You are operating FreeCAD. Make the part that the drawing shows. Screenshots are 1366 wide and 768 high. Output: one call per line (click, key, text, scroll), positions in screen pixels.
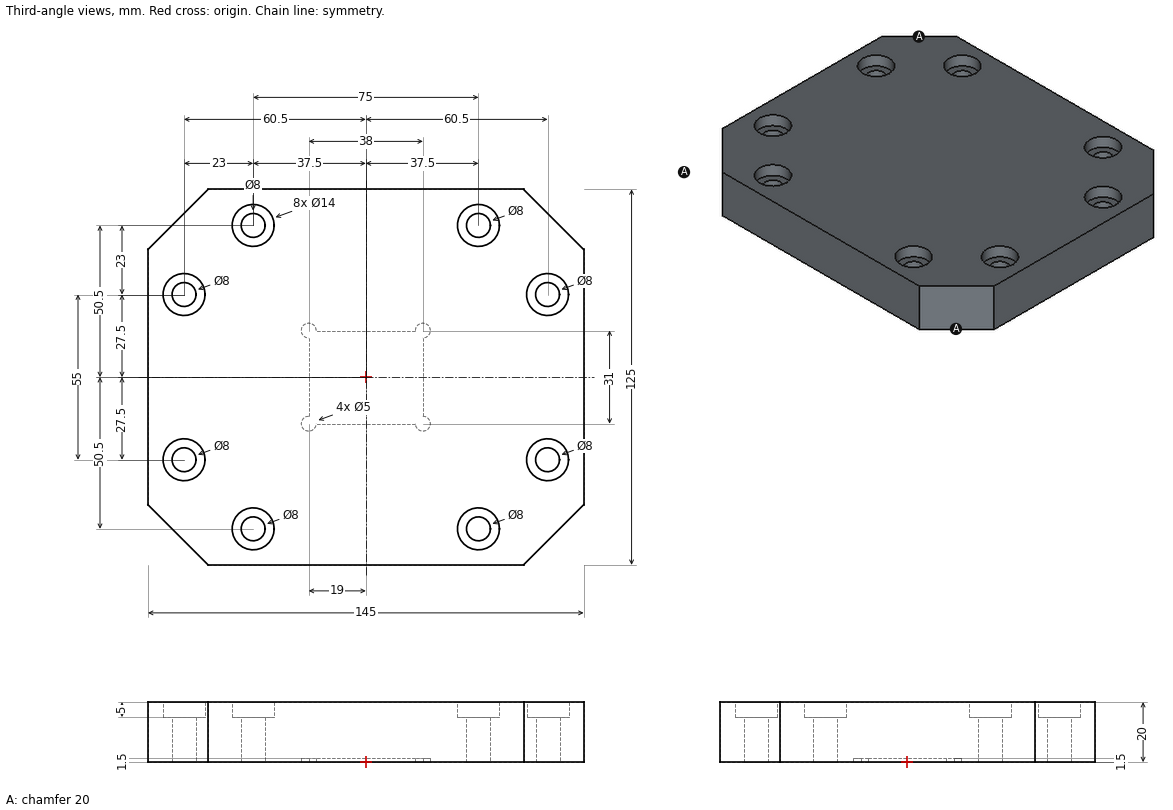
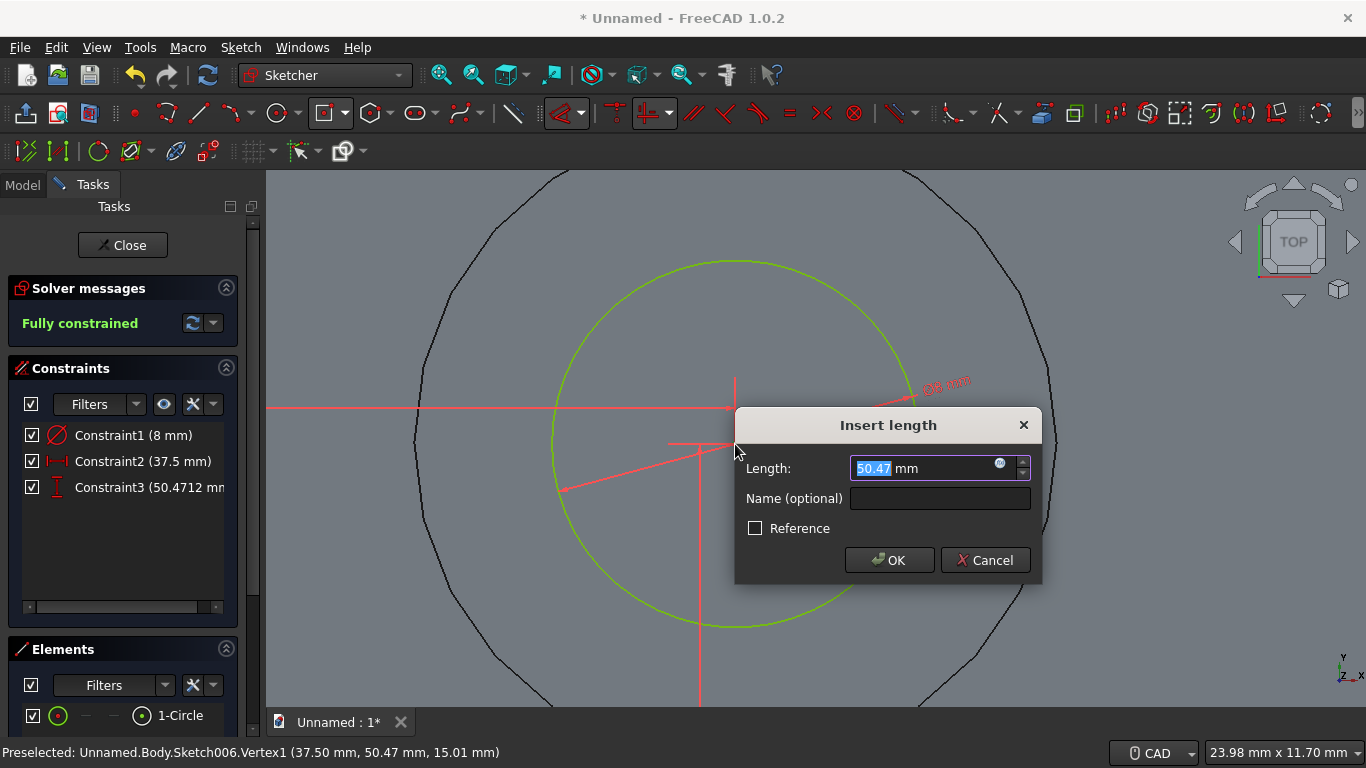
text(50.5)
key(Return)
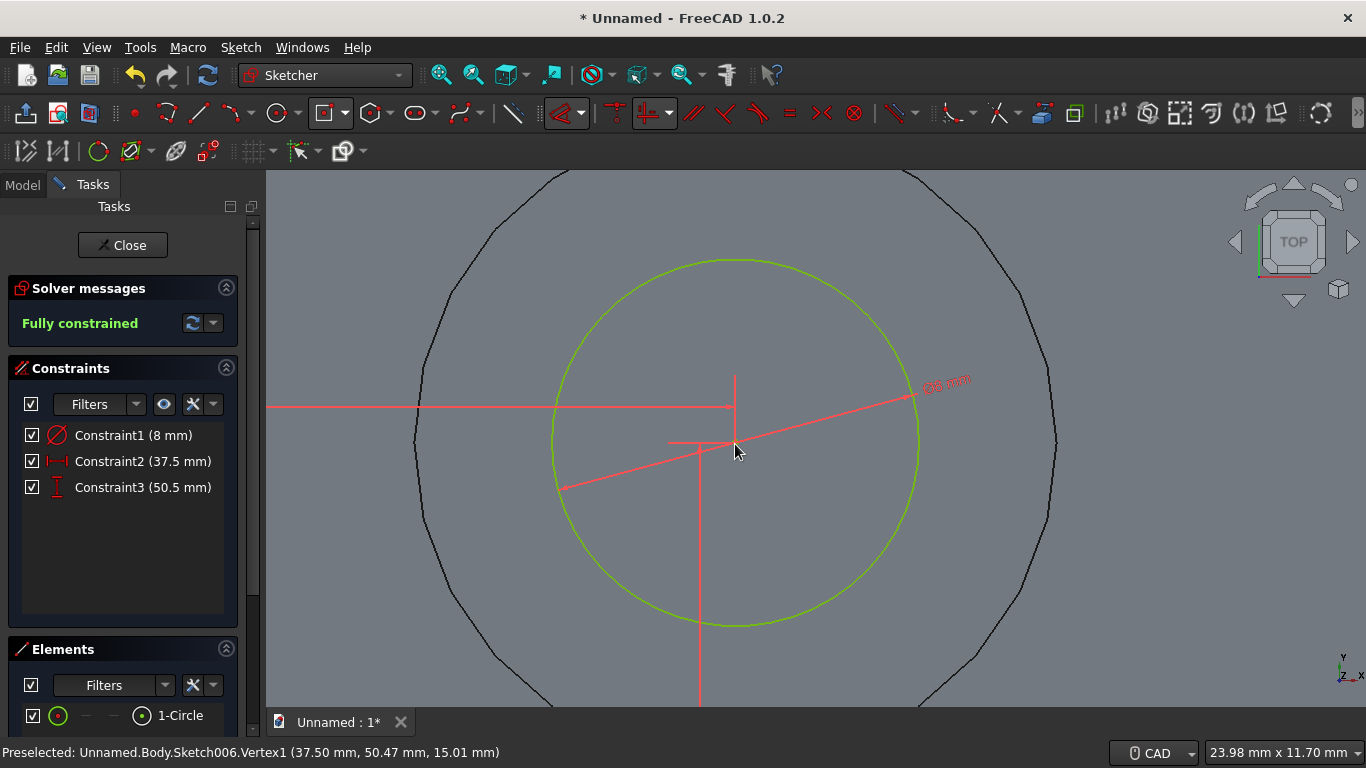
click(123, 245)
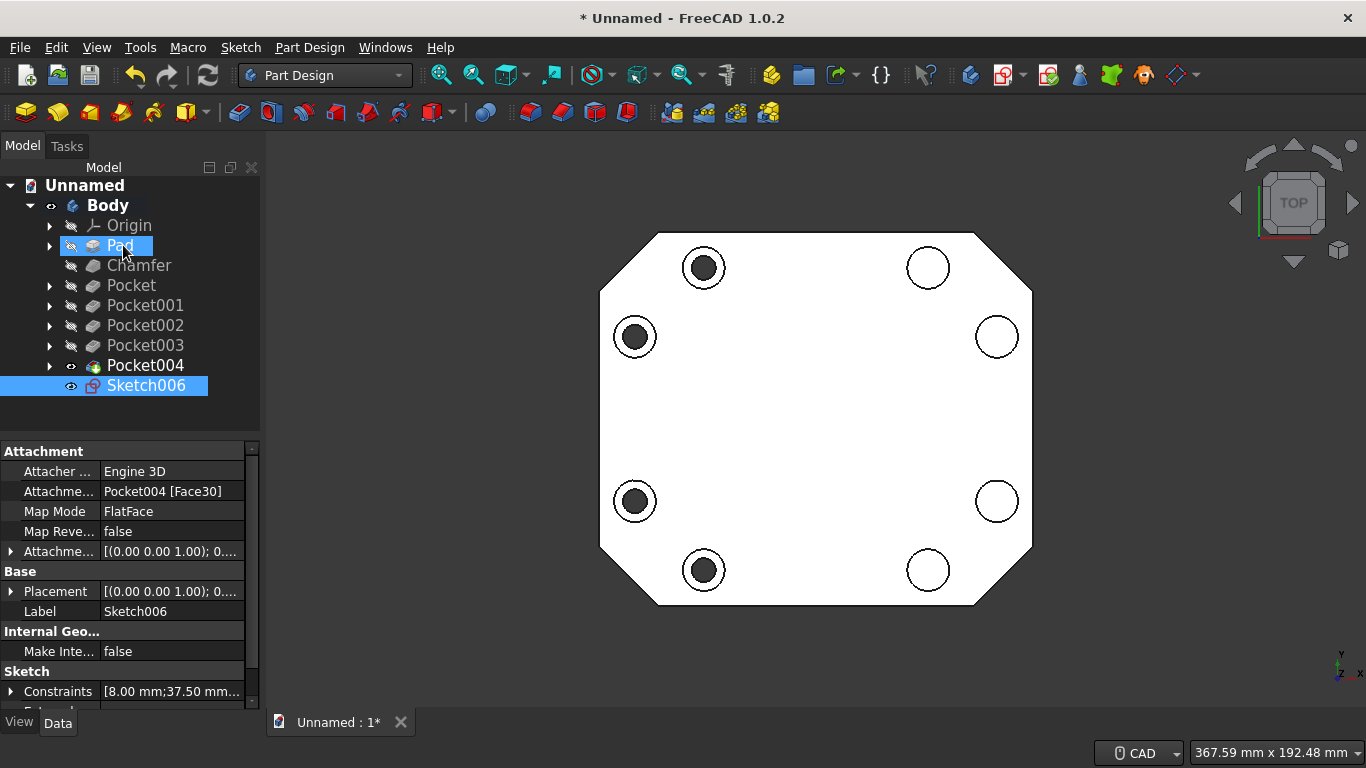
click(240, 112)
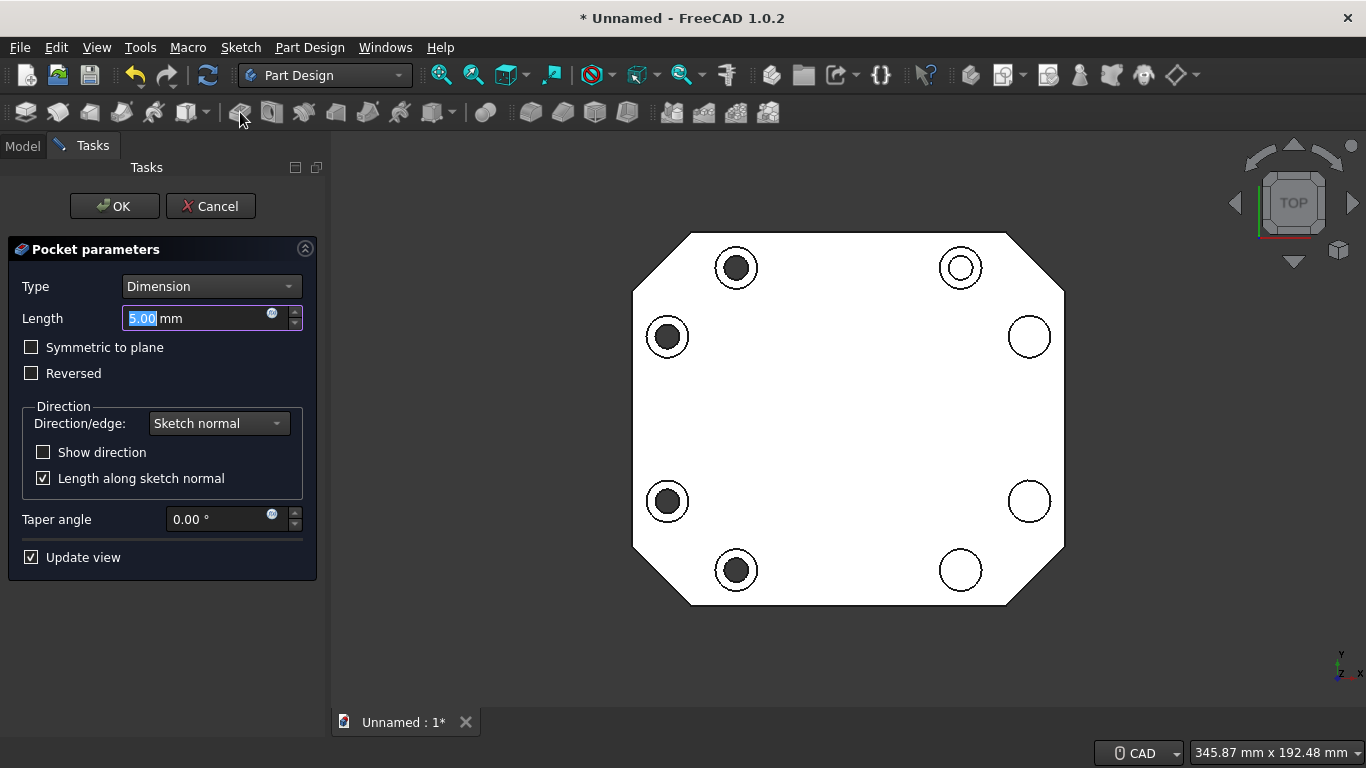
click(212, 286)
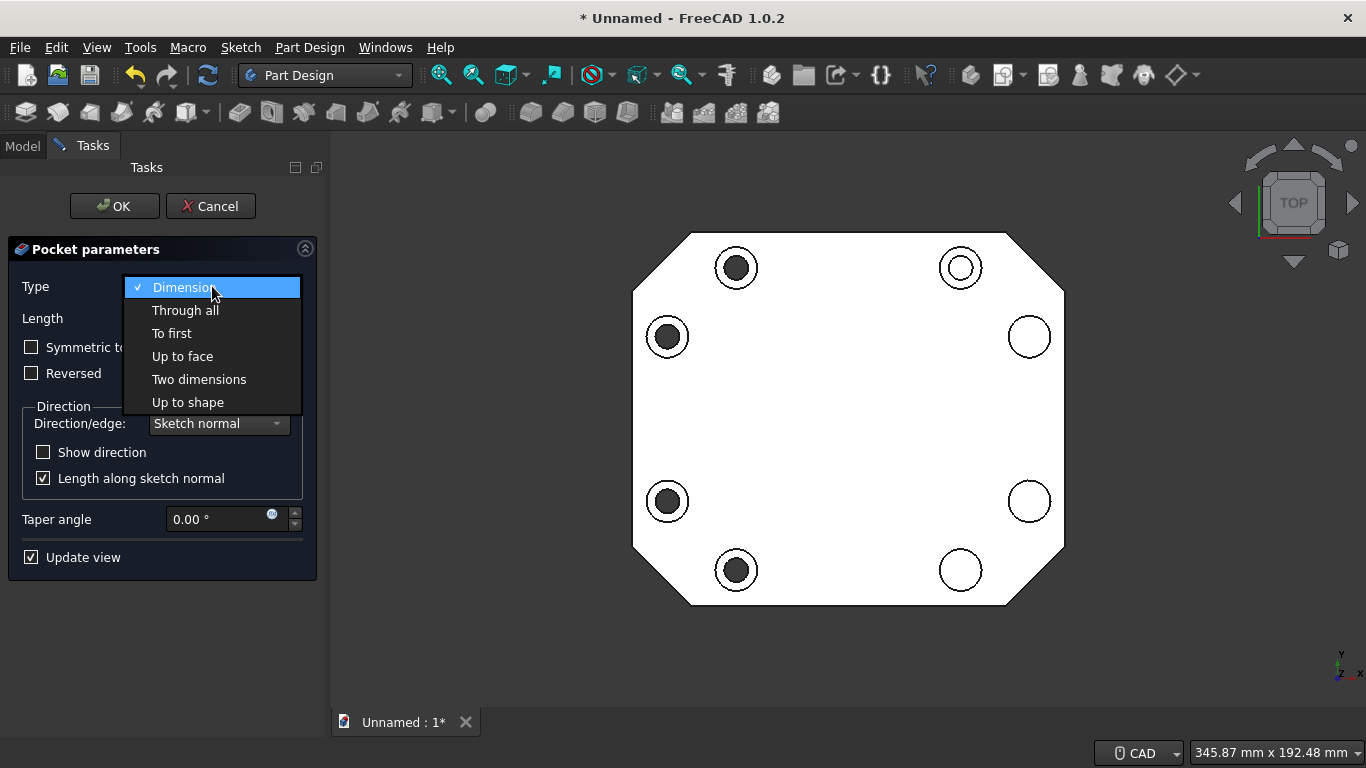
click(212, 334)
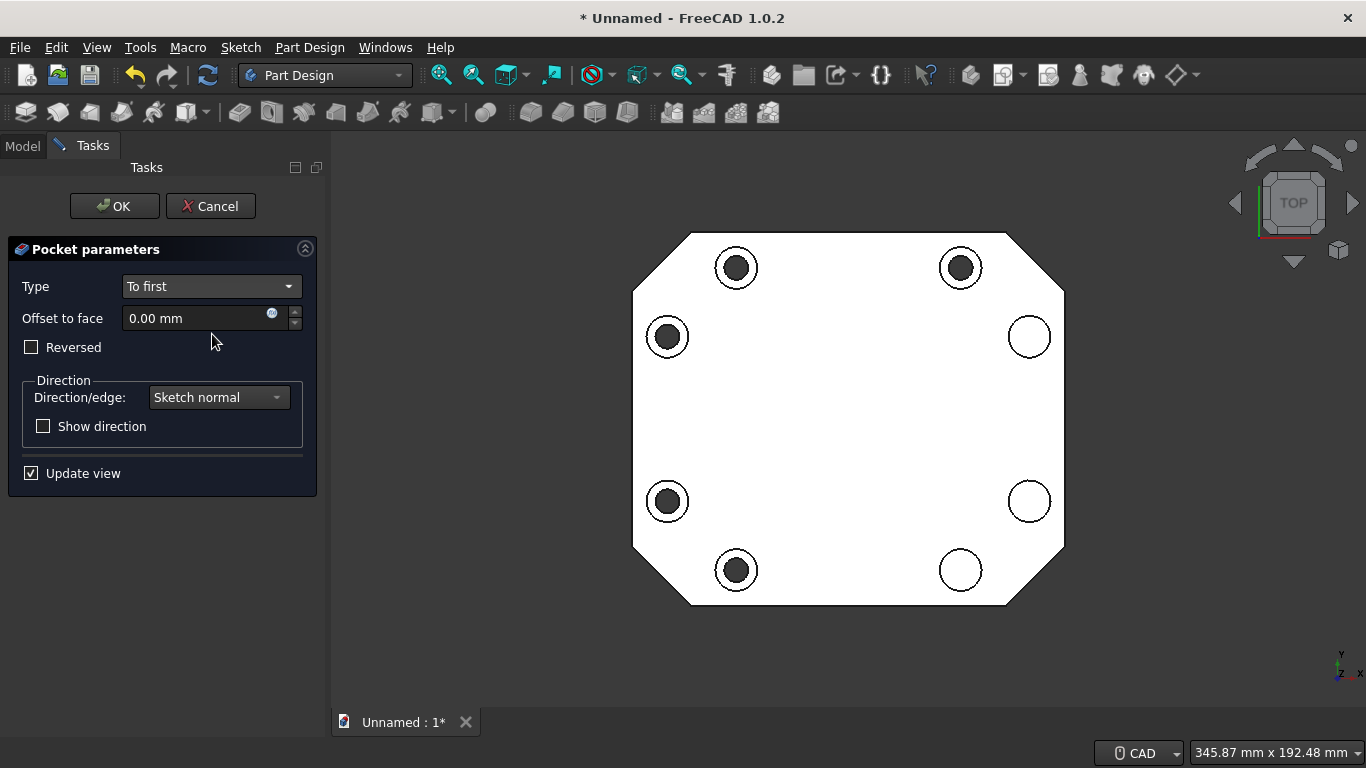
click(115, 206)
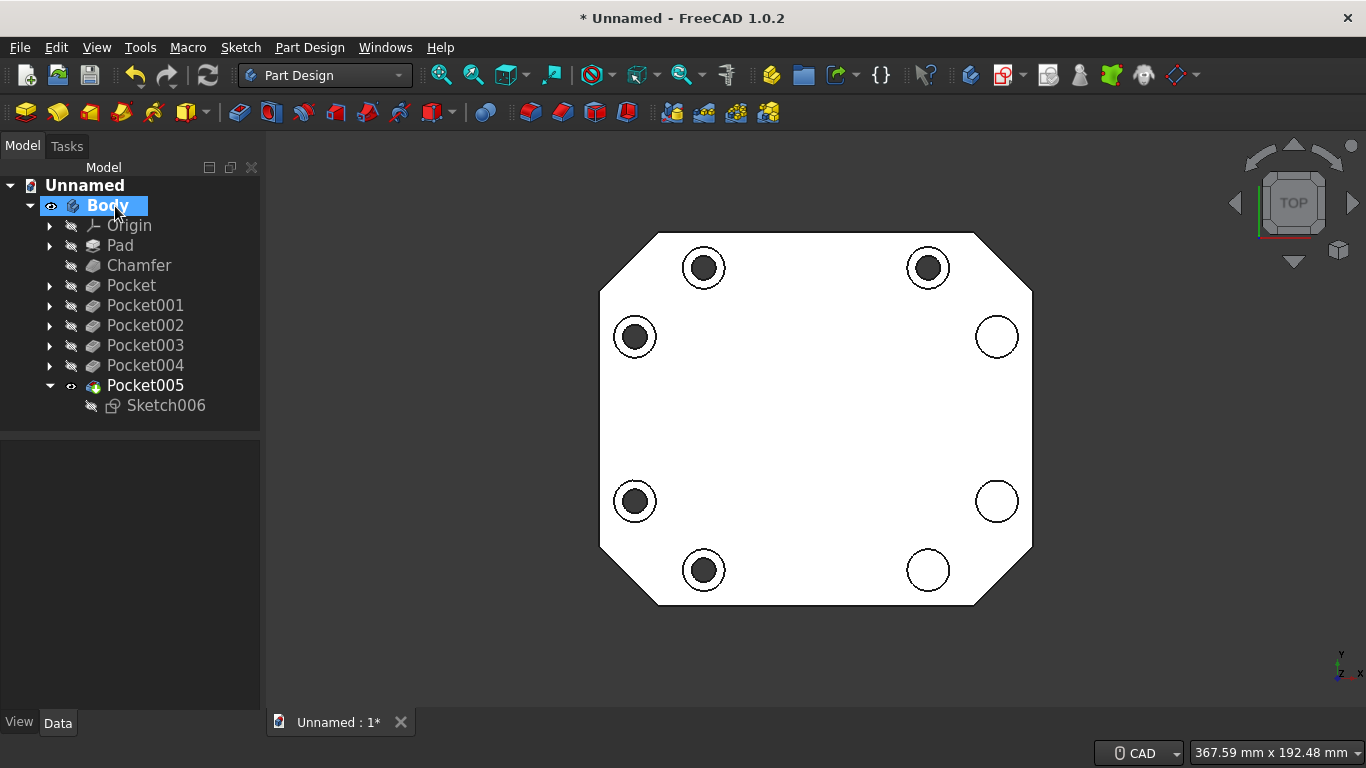
click(928, 569)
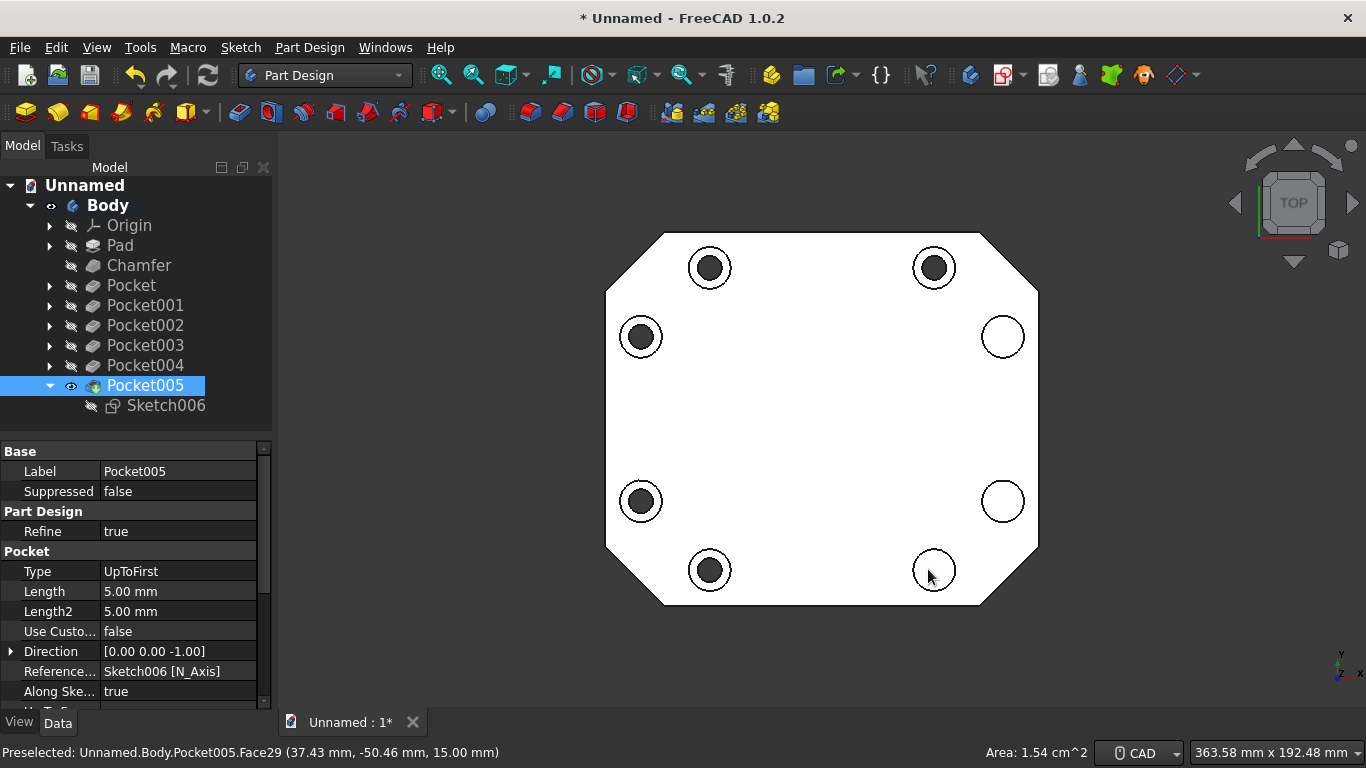
click(1004, 76)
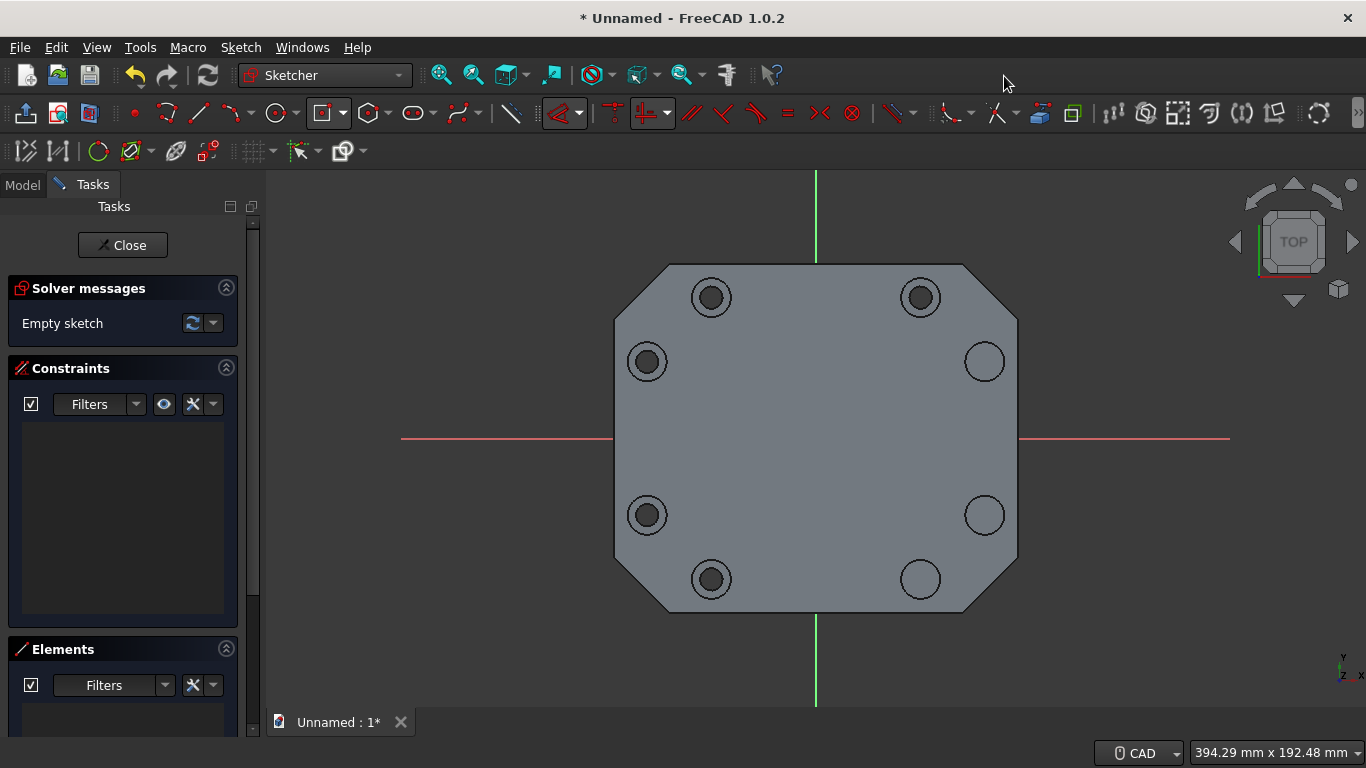
key(q)
key(s)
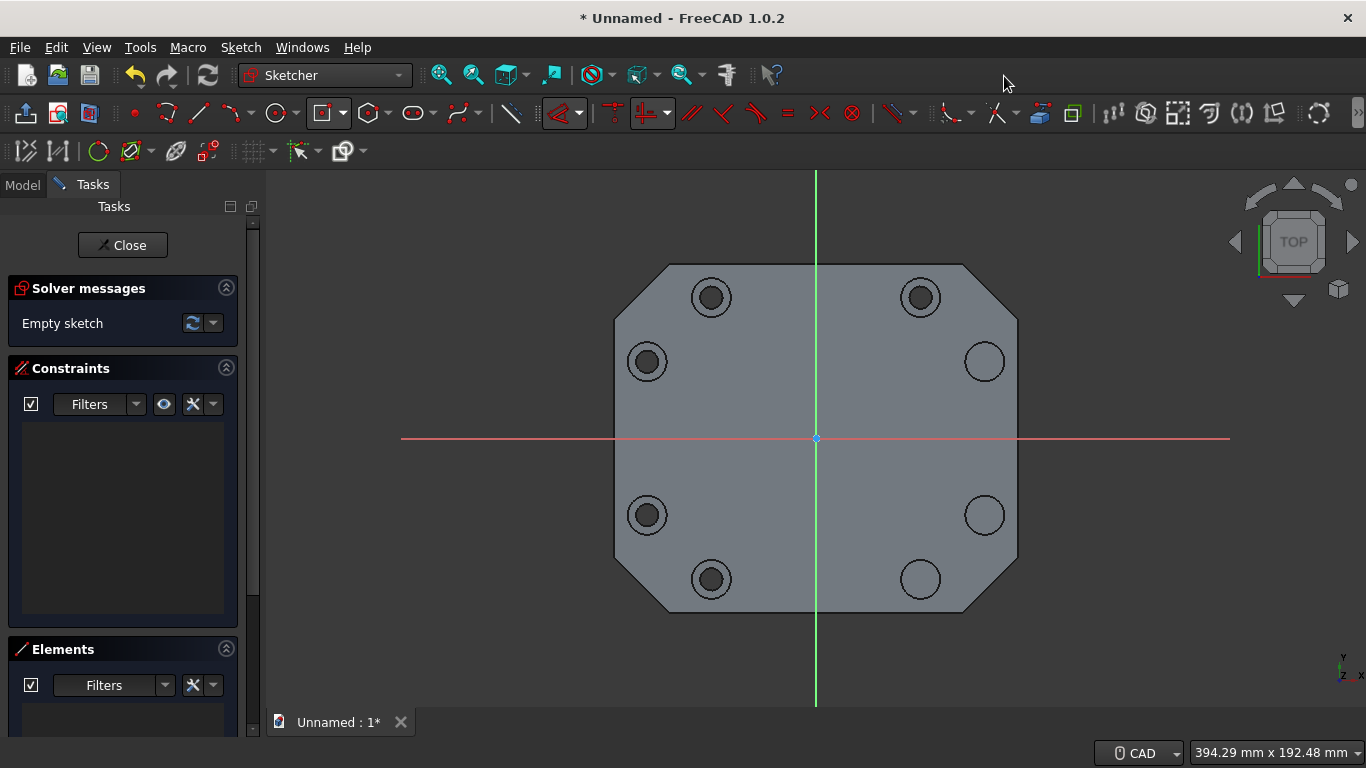
scroll(1000, 357, up, 14)